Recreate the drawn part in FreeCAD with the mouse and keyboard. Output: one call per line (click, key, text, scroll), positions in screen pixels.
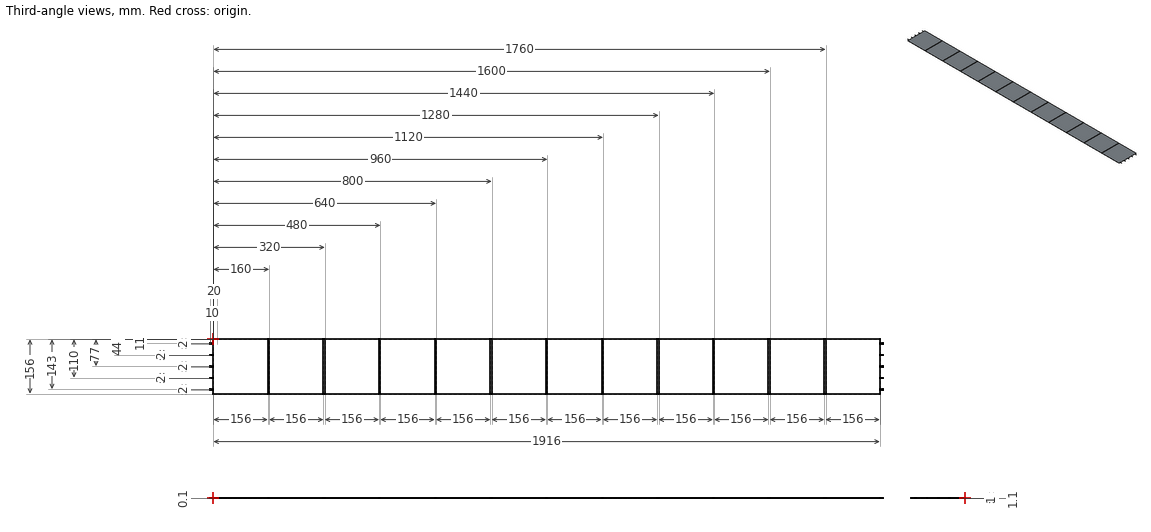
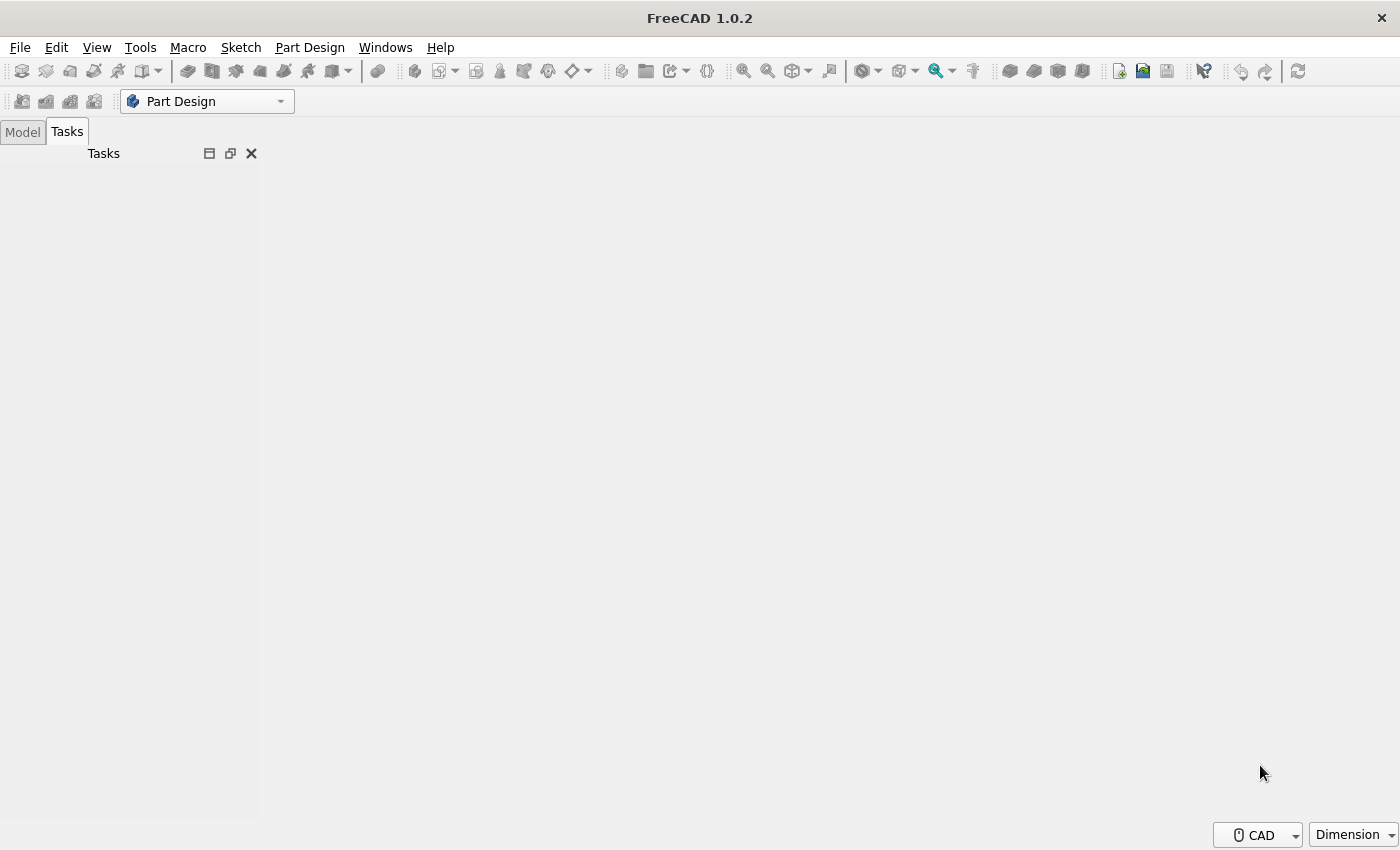
click(1120, 72)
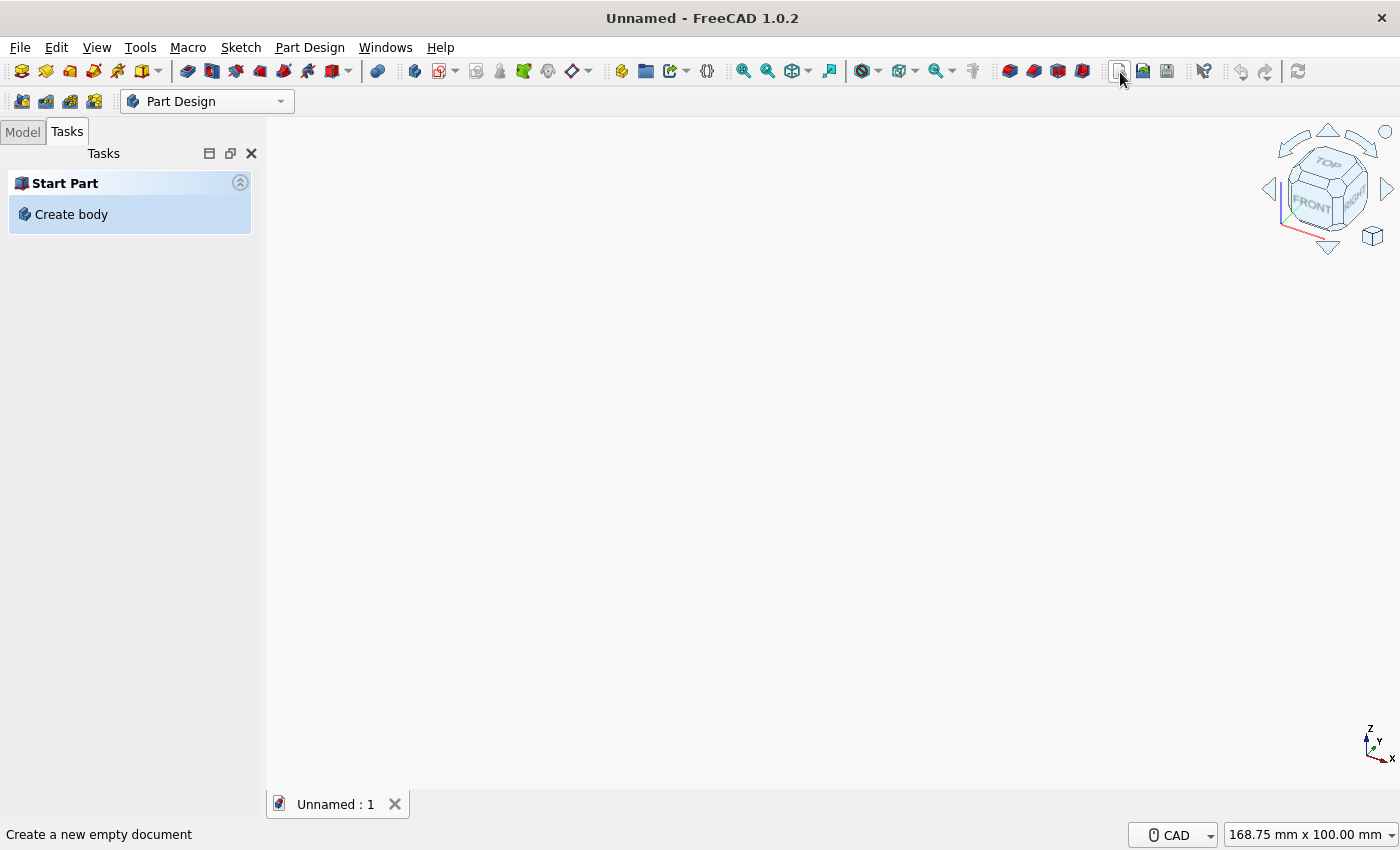
click(440, 72)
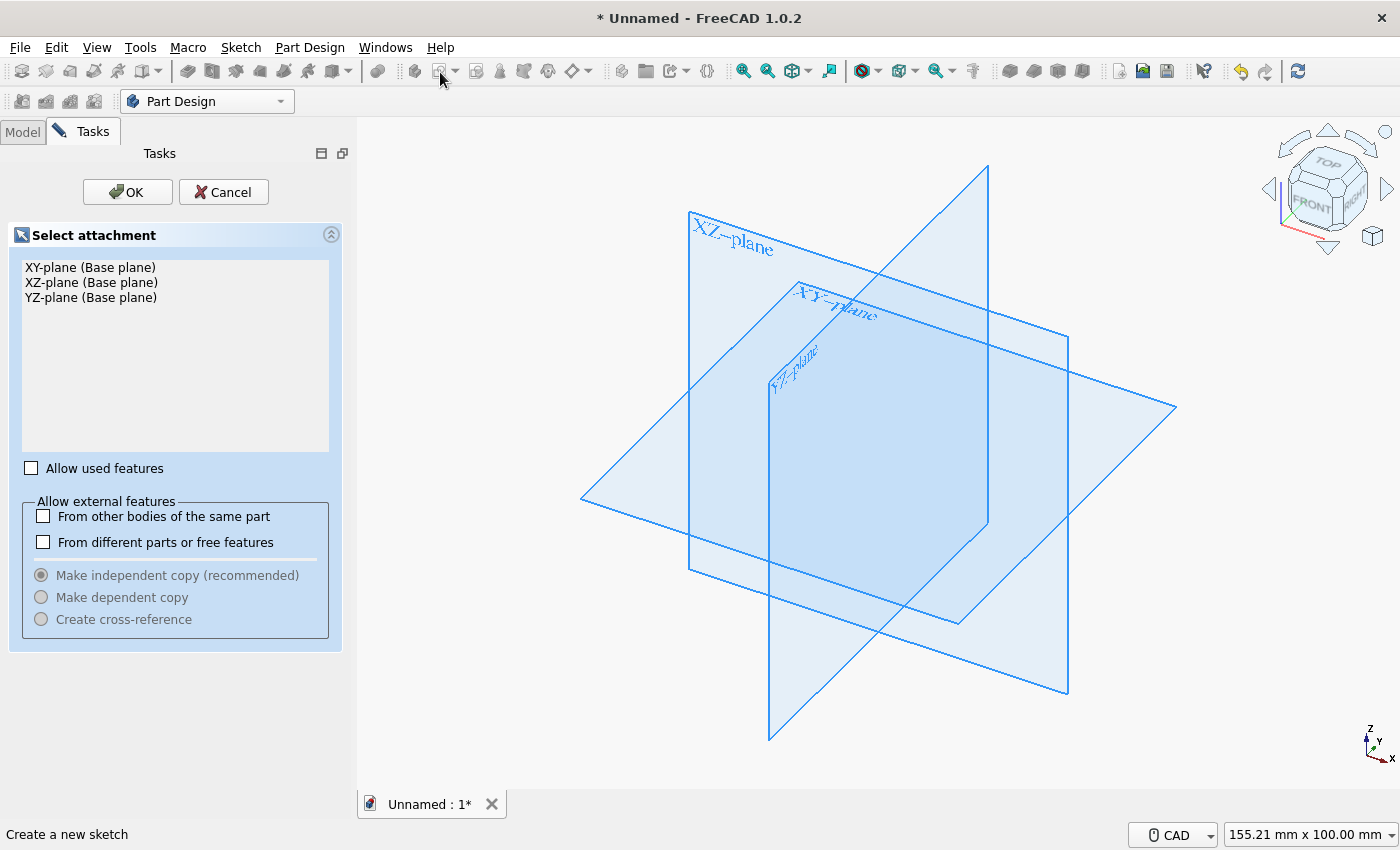
click(82, 268)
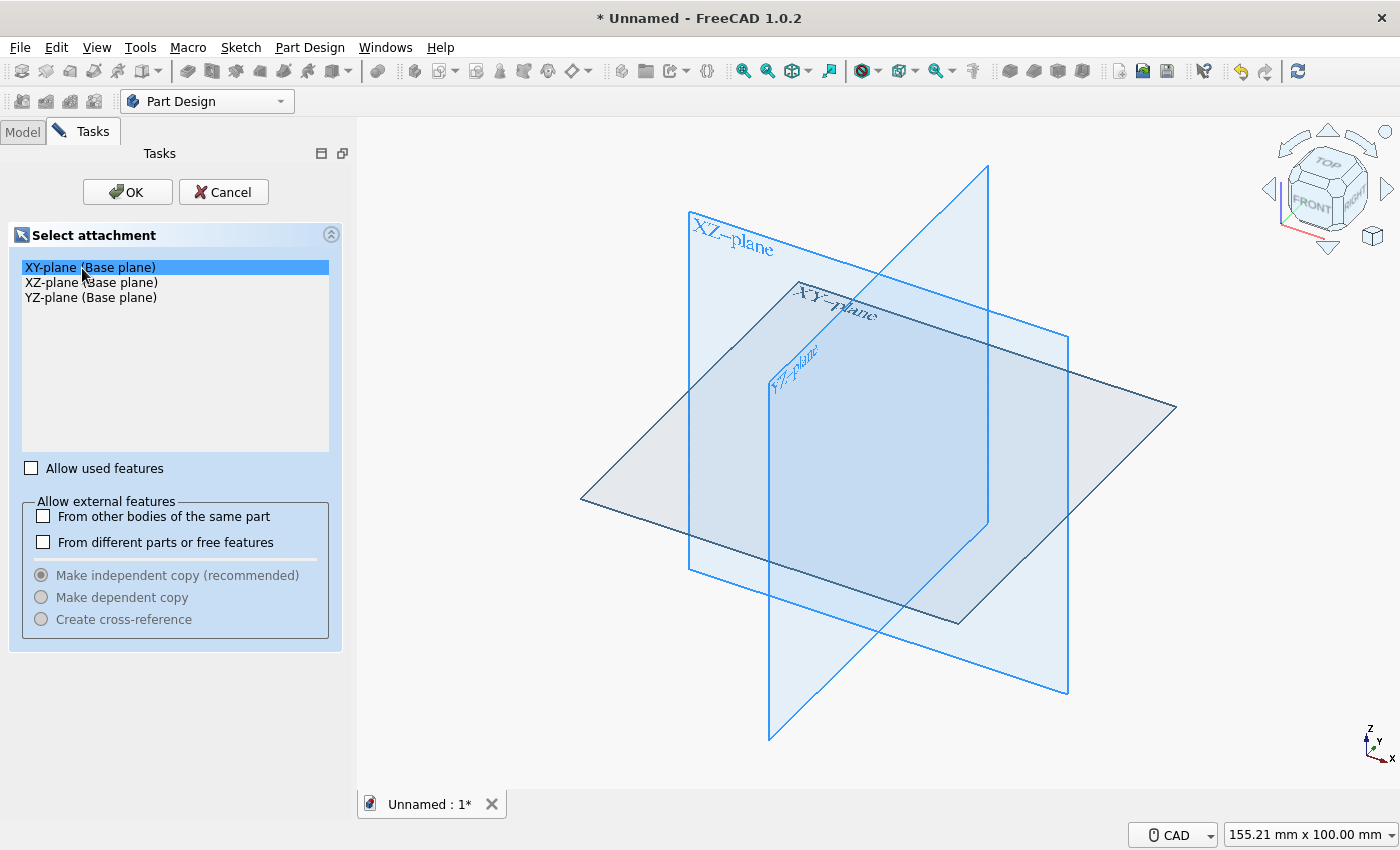
click(128, 192)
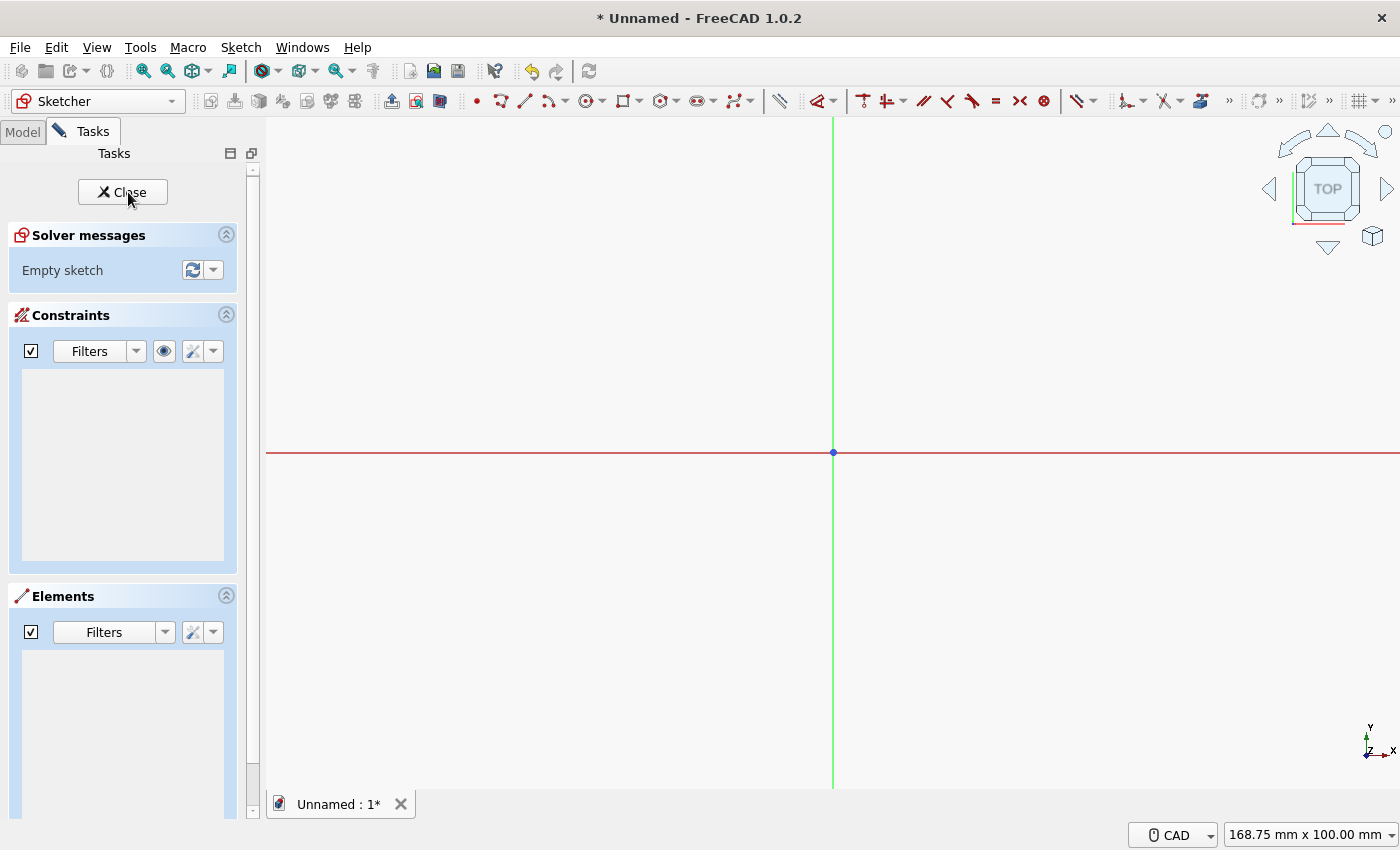
scroll(424, 426, down, 15)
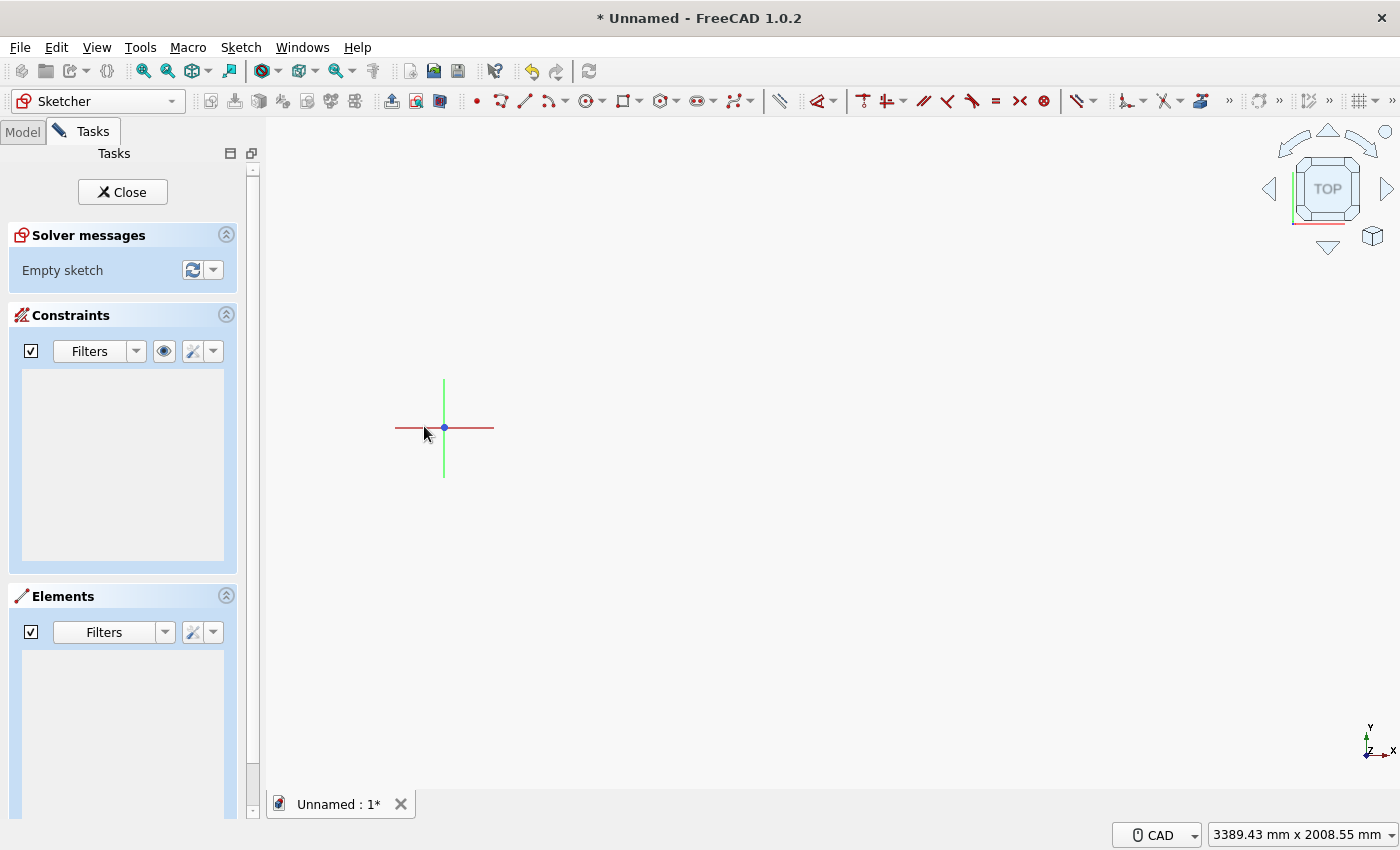
key(g)
key(r)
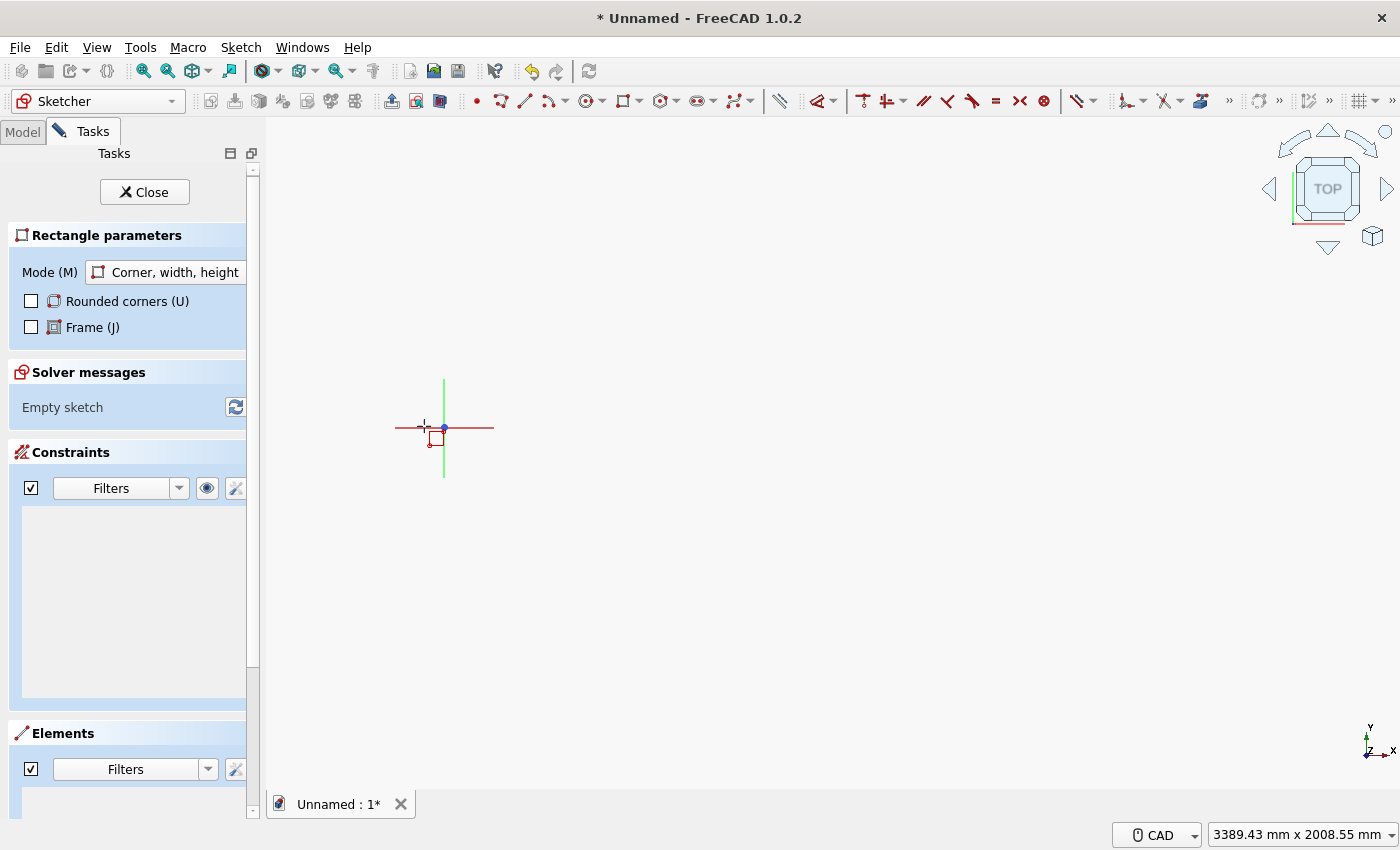
click(444, 428)
click(1086, 480)
key(Escape)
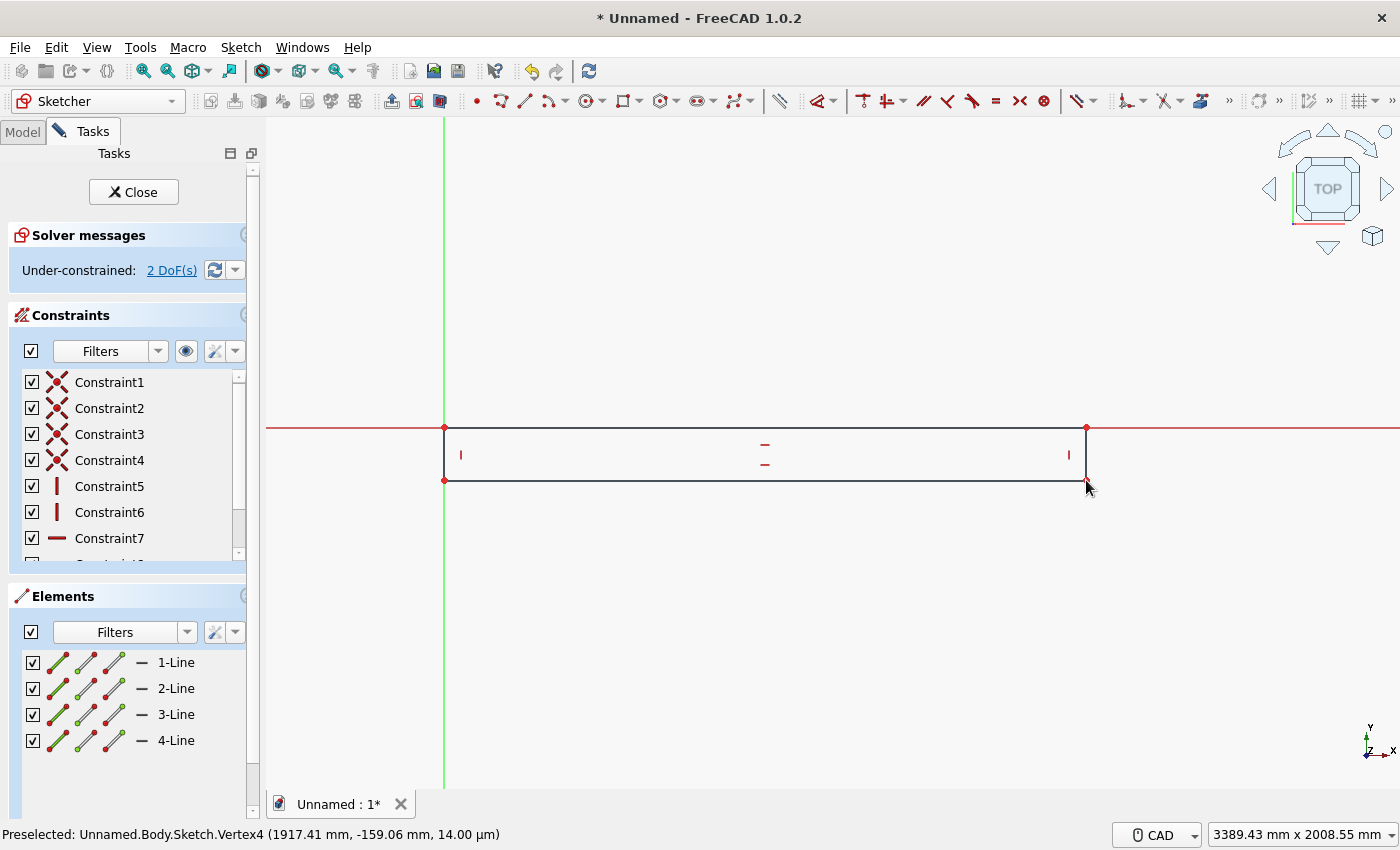
click(818, 102)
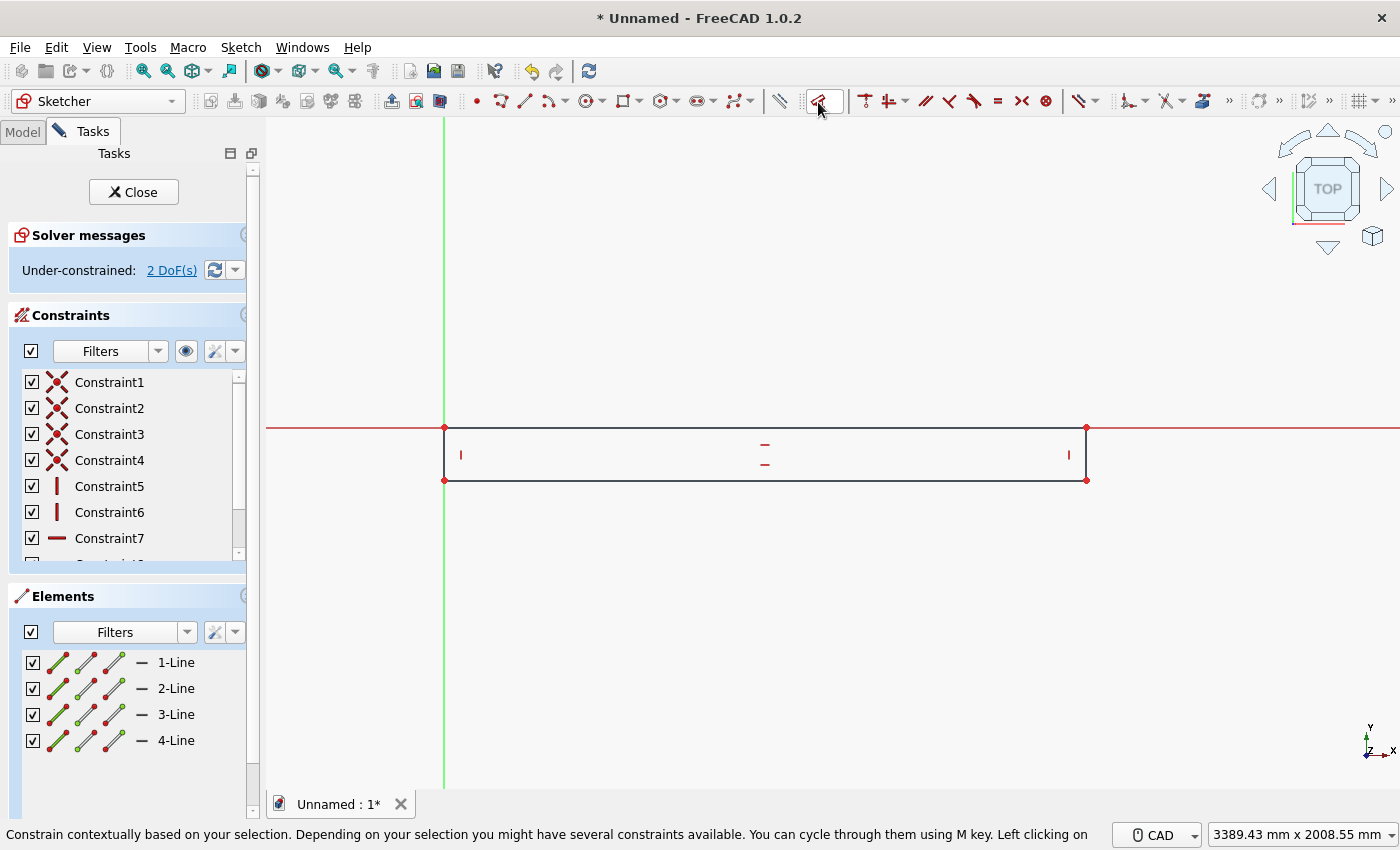
click(444, 444)
click(410, 454)